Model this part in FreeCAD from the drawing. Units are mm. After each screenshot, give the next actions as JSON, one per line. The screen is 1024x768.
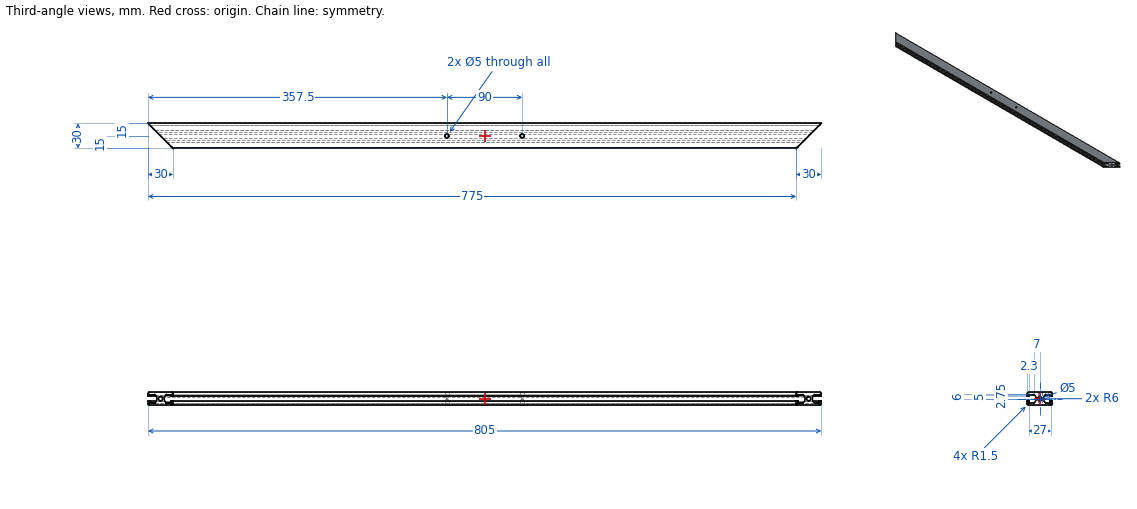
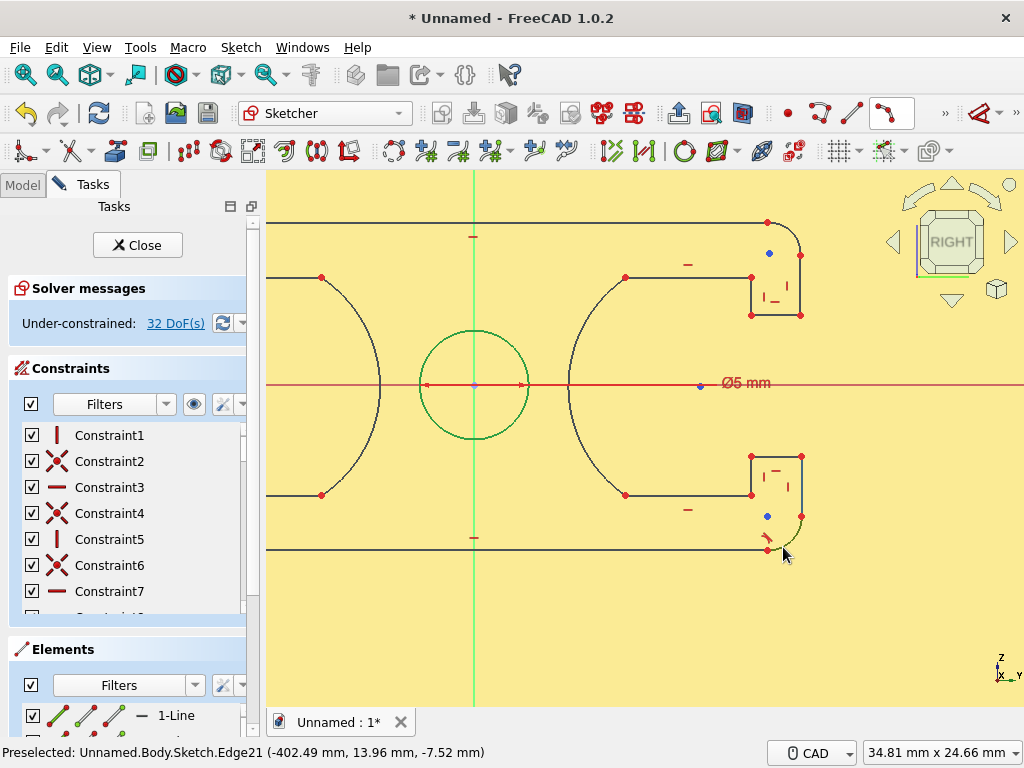
{"action": "key", "text": "t"}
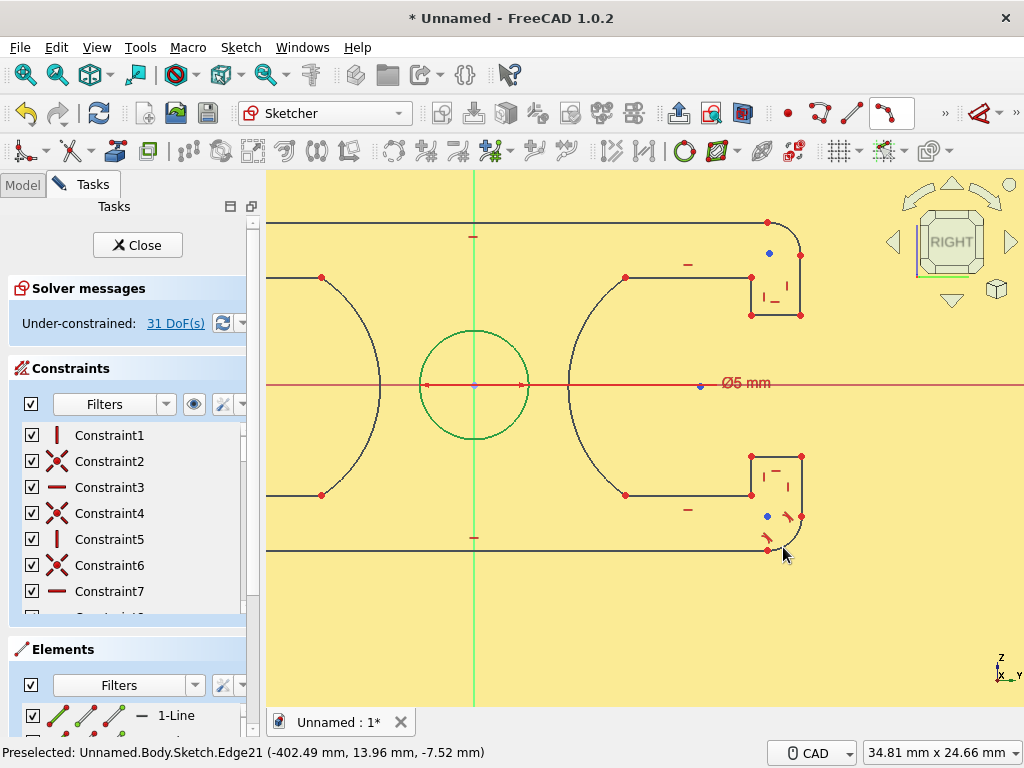
{"action": "left_click", "coordinate": [800, 297]}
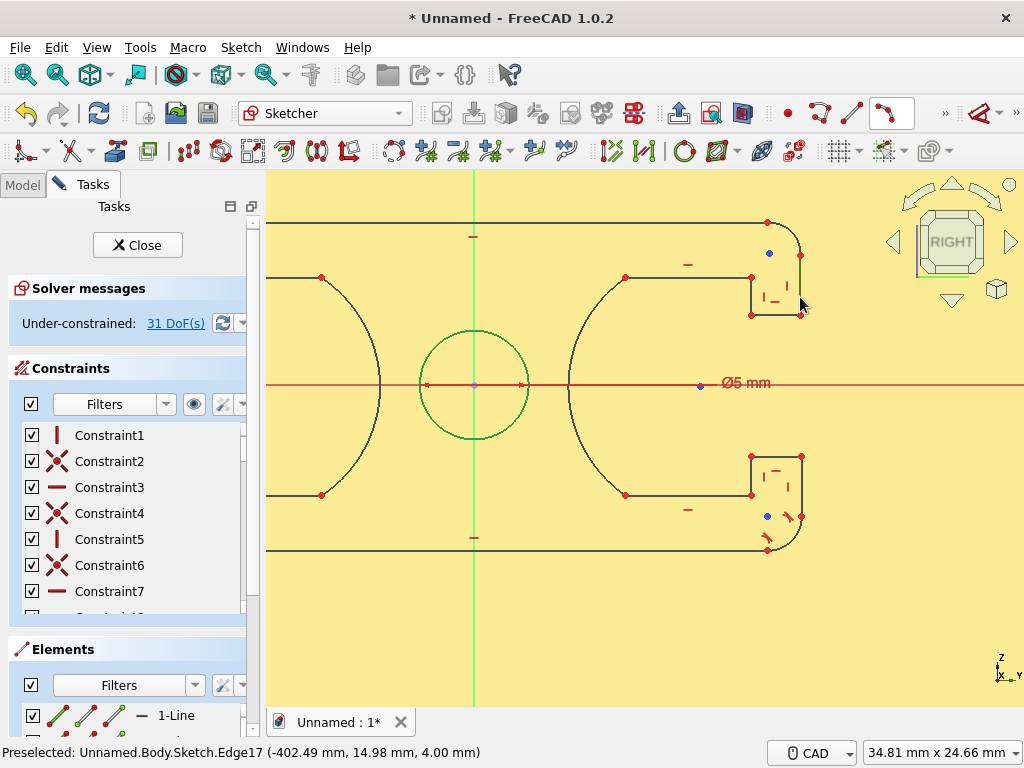
{"action": "left_click", "coordinate": [797, 240]}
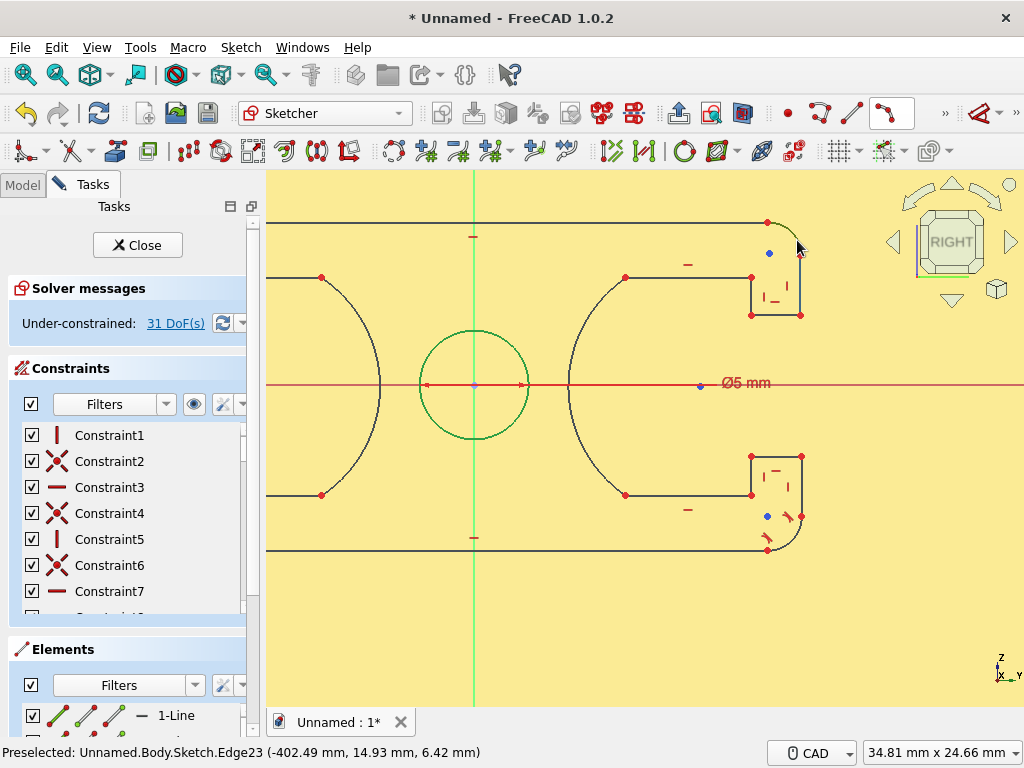
{"action": "key", "text": "t"}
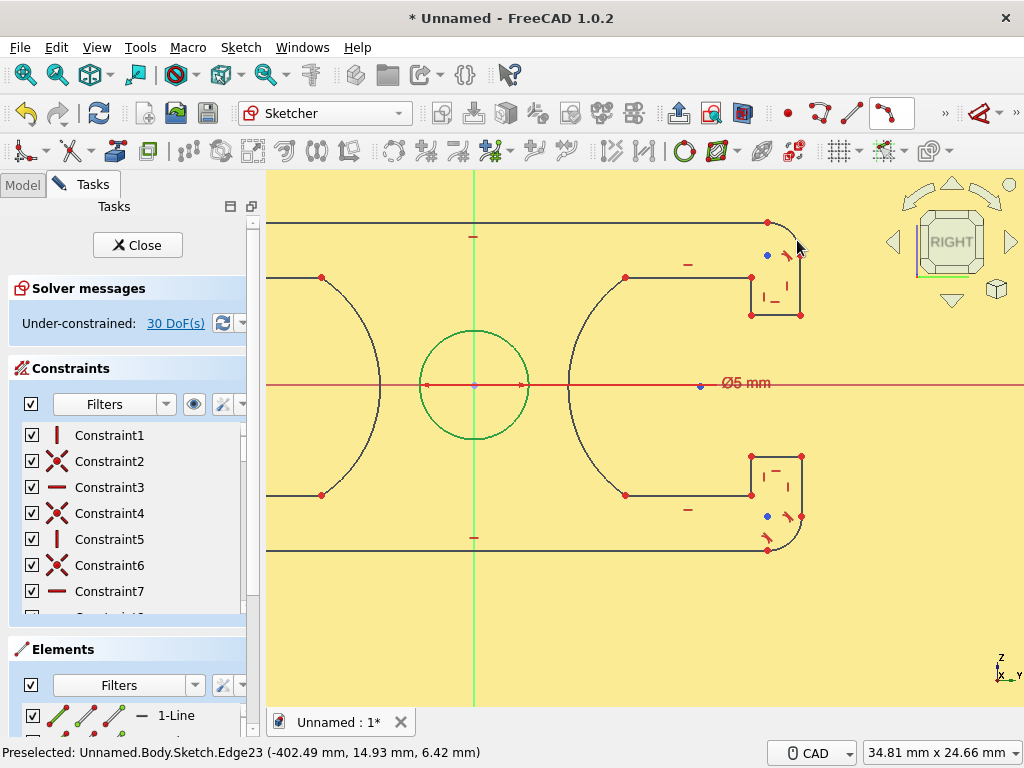
{"action": "left_click", "coordinate": [591, 223]}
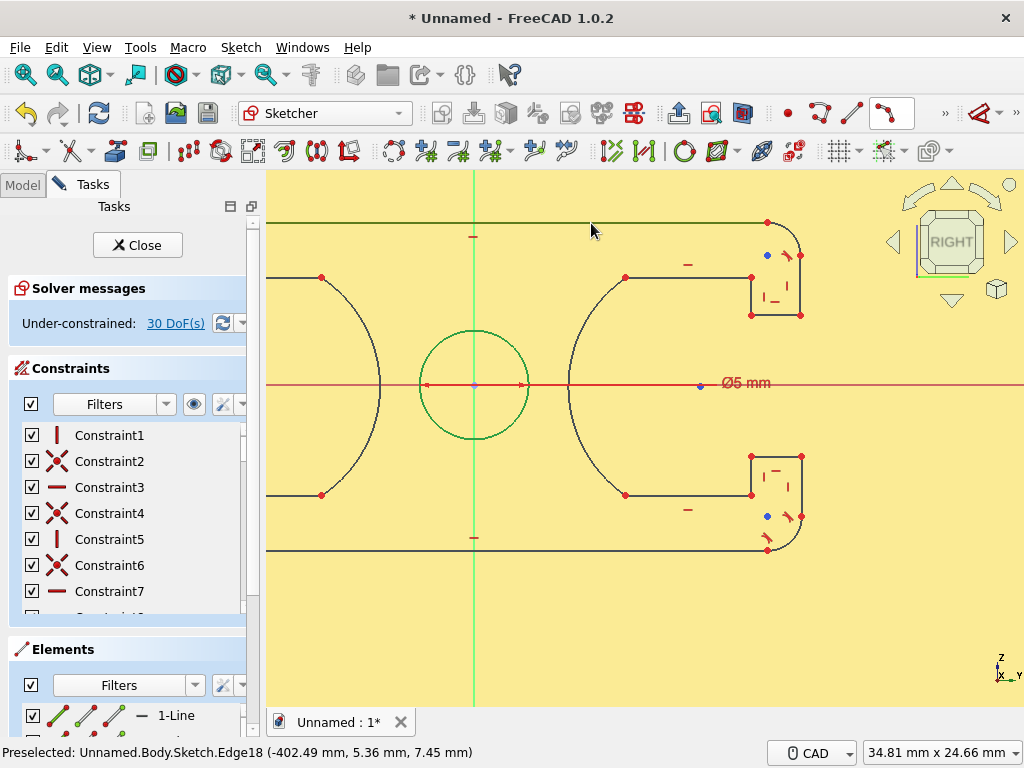
{"action": "left_click", "coordinate": [797, 241]}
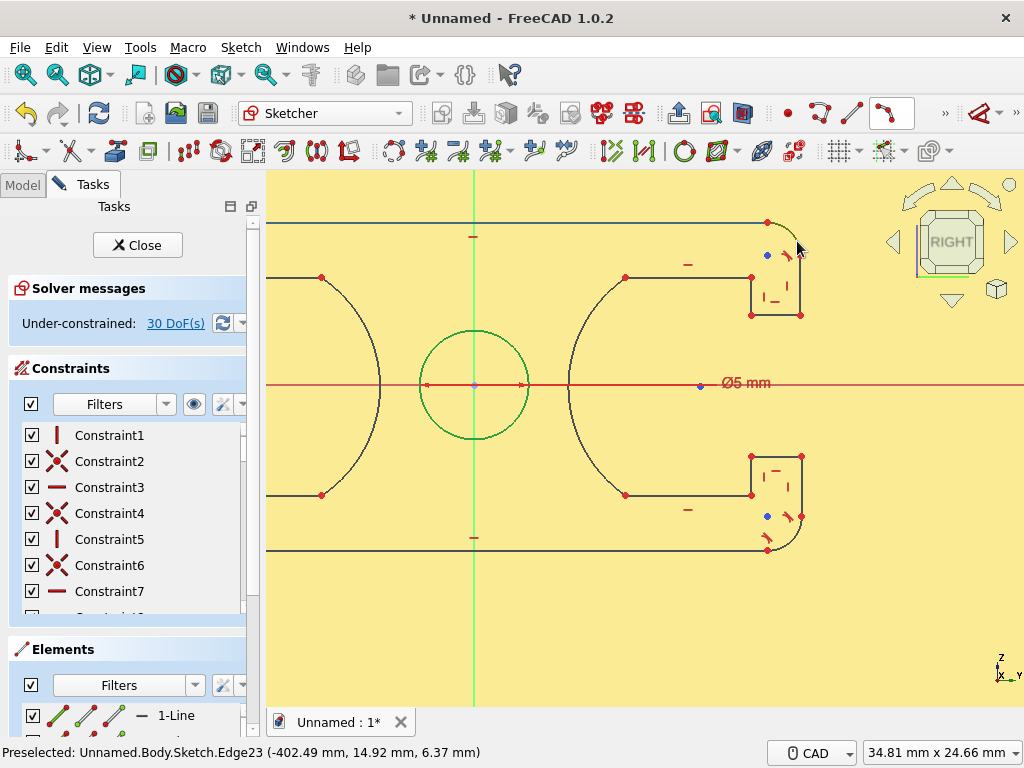
{"action": "key", "text": "t"}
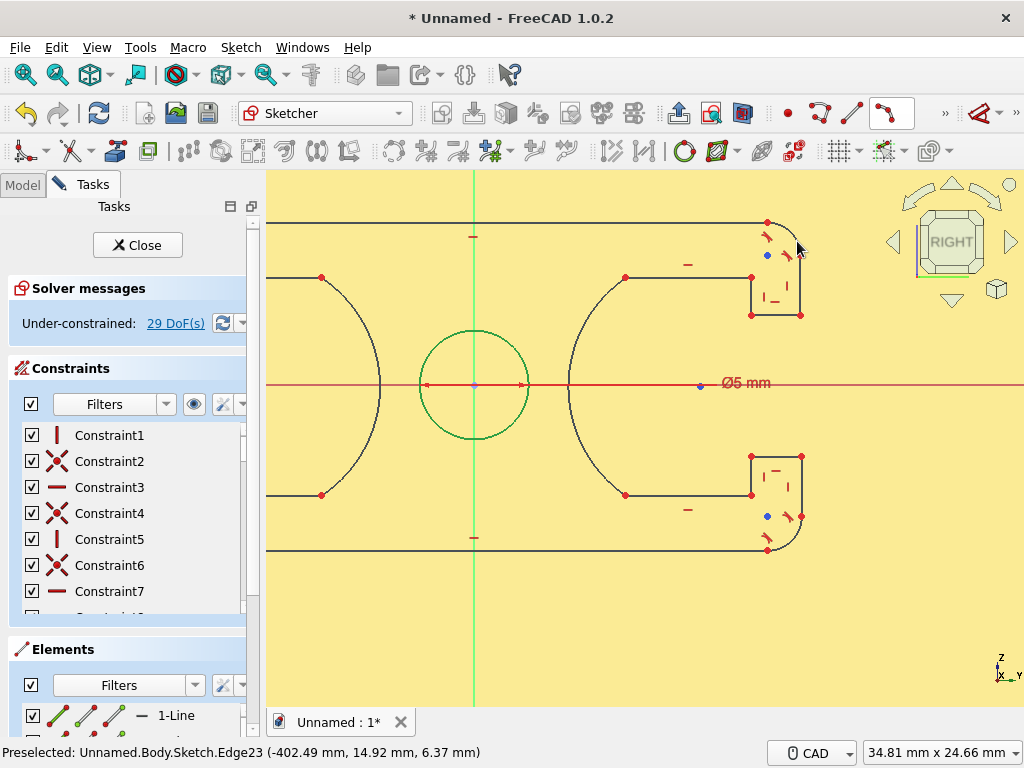
{"action": "left_click", "coordinate": [591, 223]}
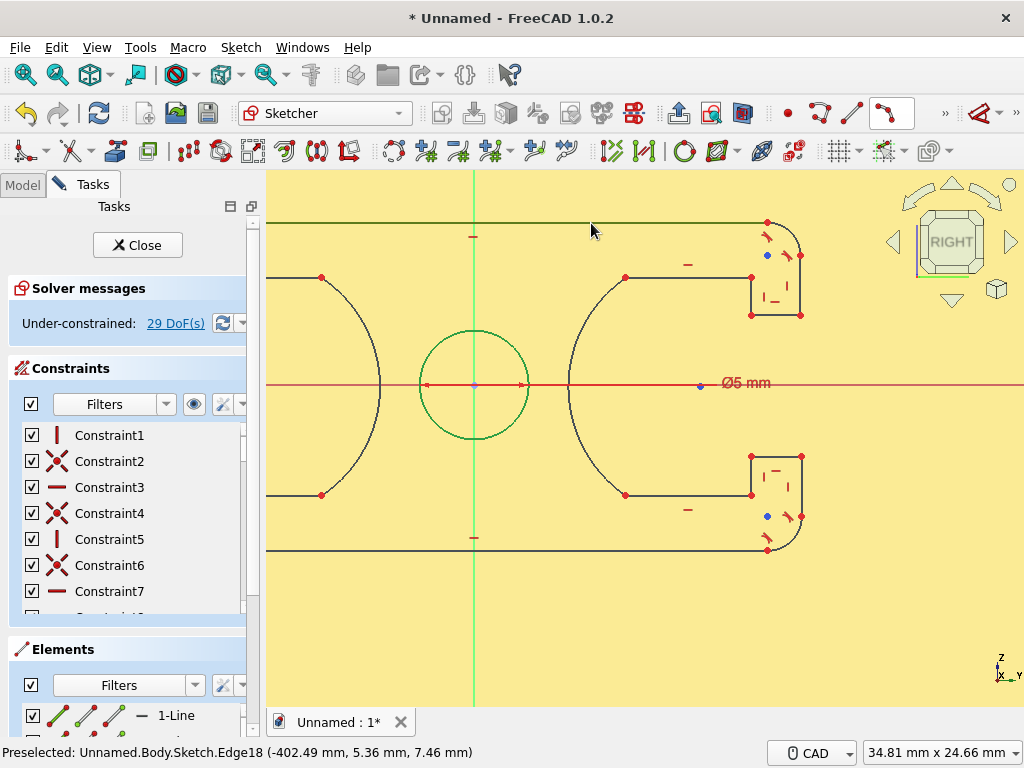
{"action": "scroll", "coordinate": [784, 547], "scroll_direction": "down", "scroll_amount": 2}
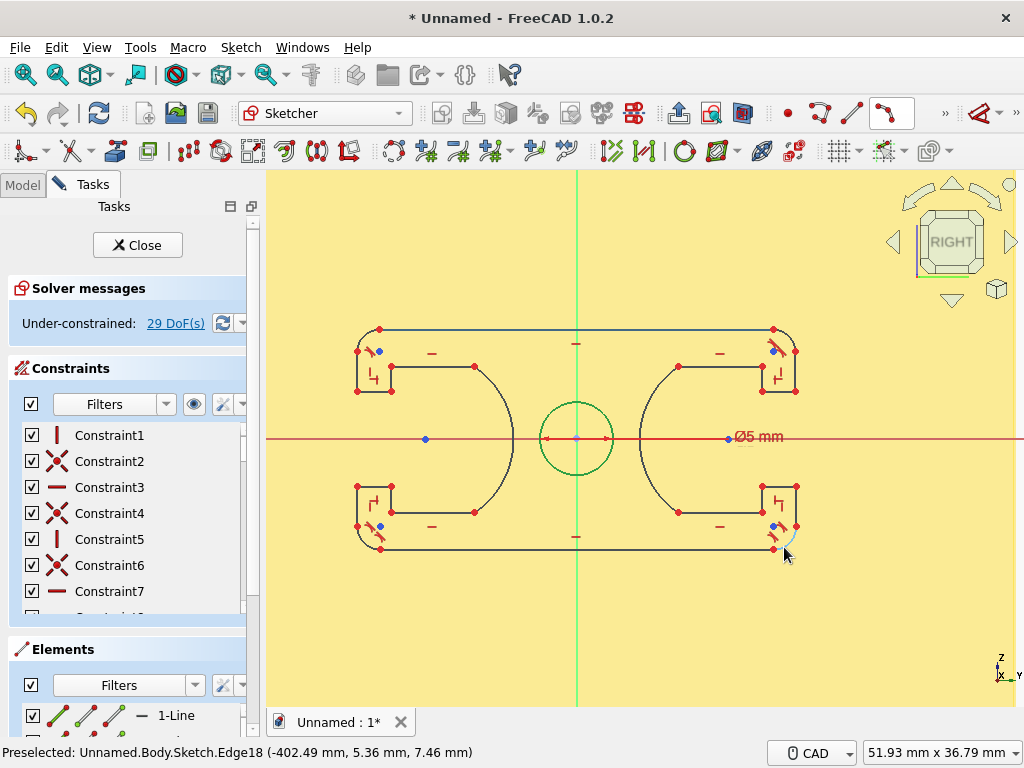
{"action": "scroll", "coordinate": [369, 332], "scroll_direction": "up", "scroll_amount": 2}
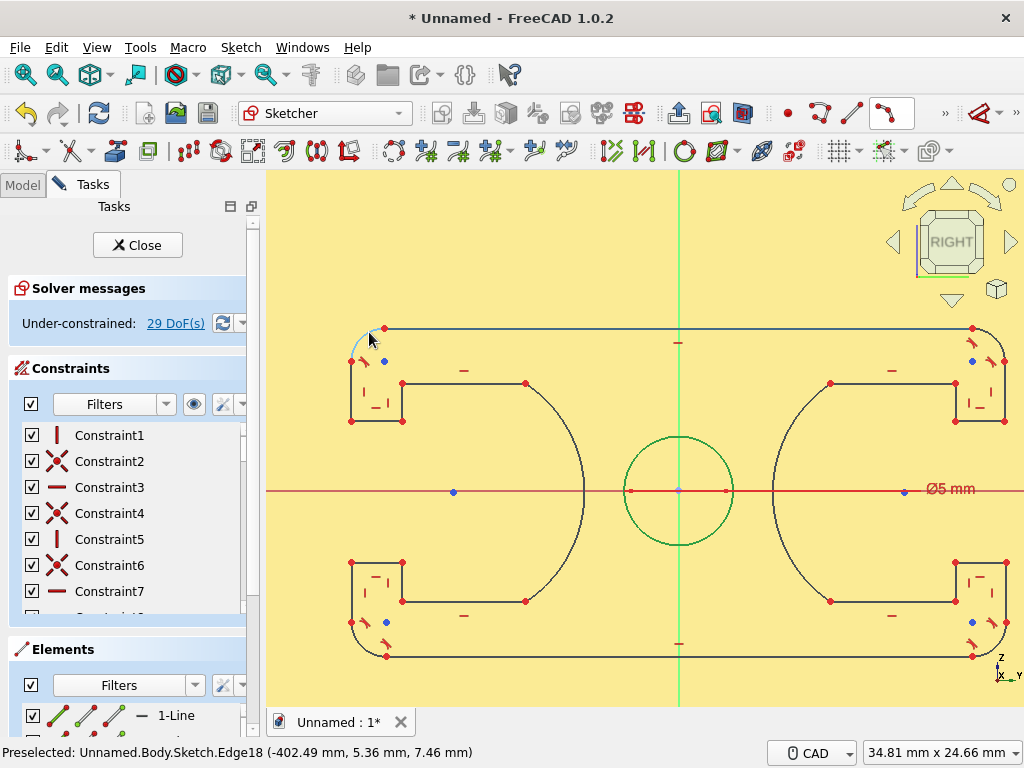
{"action": "left_click", "coordinate": [369, 332]}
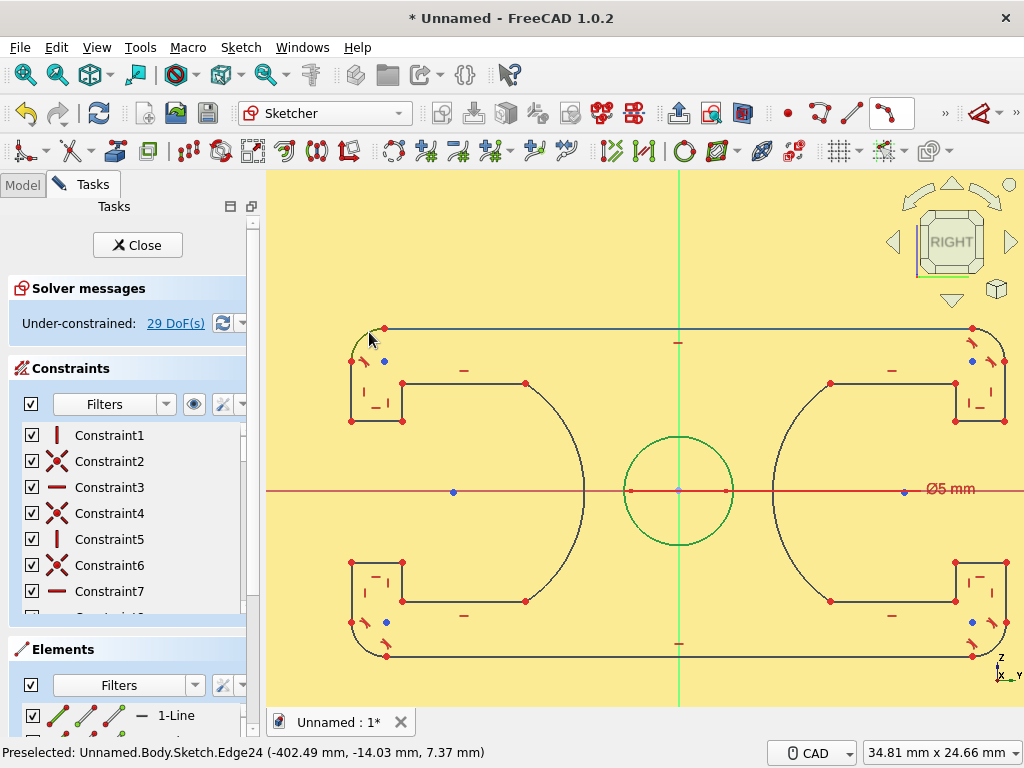
{"action": "key", "text": "t"}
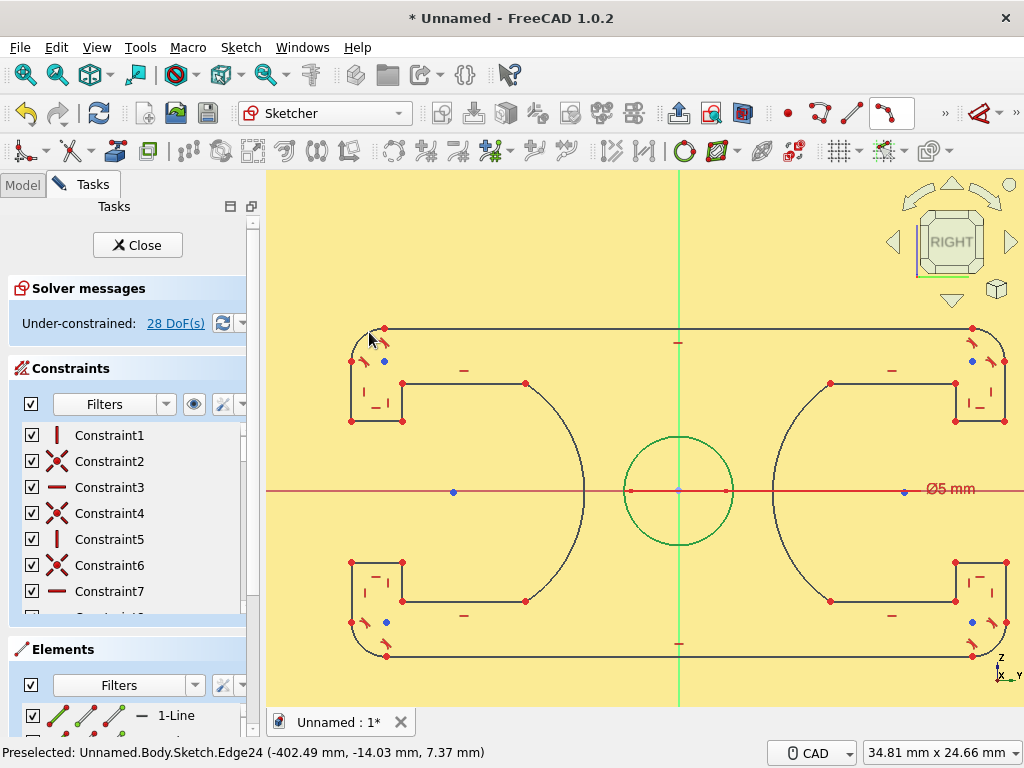
{"action": "left_click", "coordinate": [355, 638]}